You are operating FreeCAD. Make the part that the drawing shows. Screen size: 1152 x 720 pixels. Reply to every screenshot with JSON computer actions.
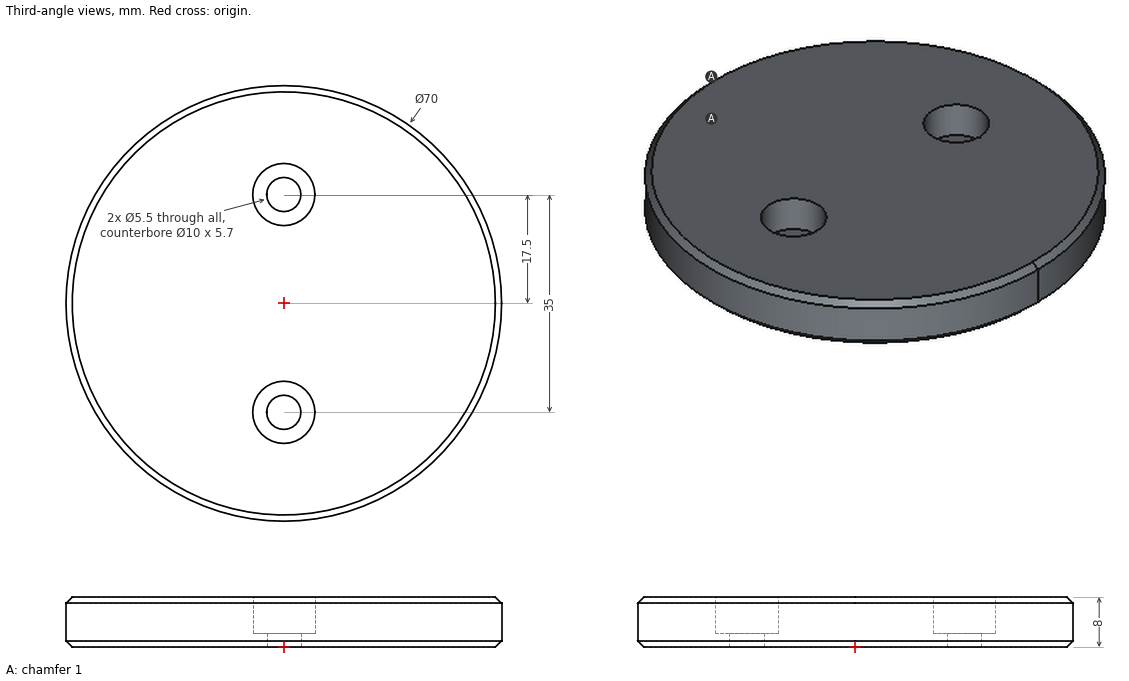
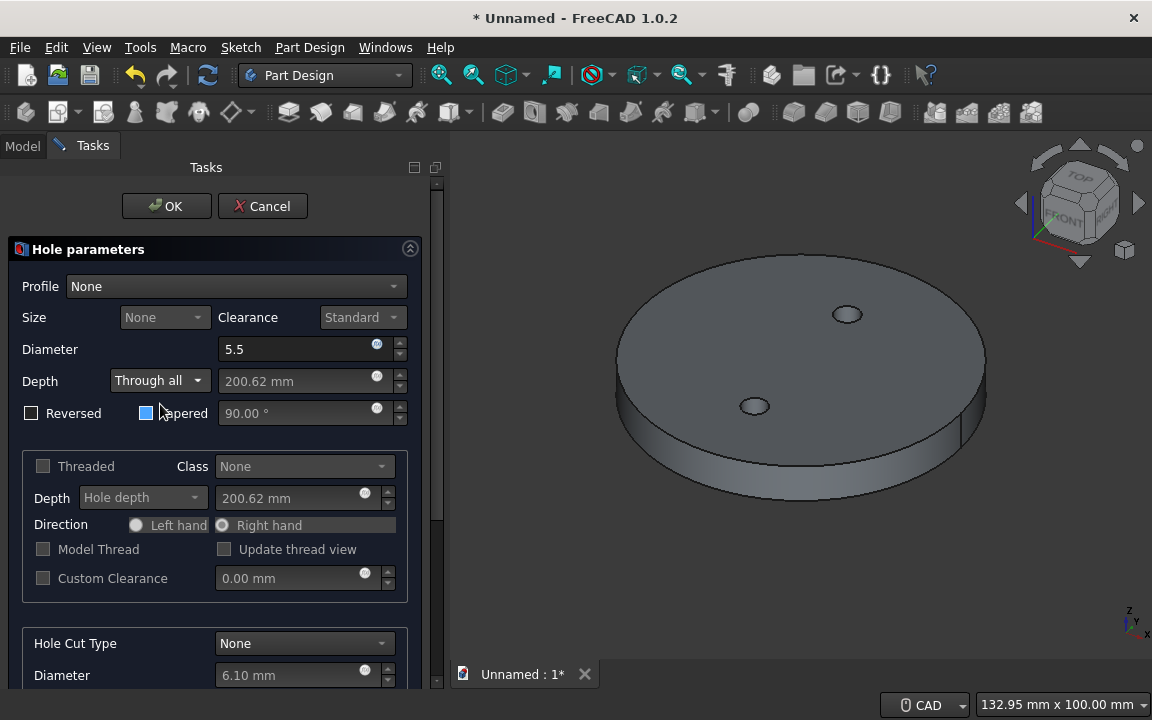
{"action": "left_click", "coordinate": [306, 644]}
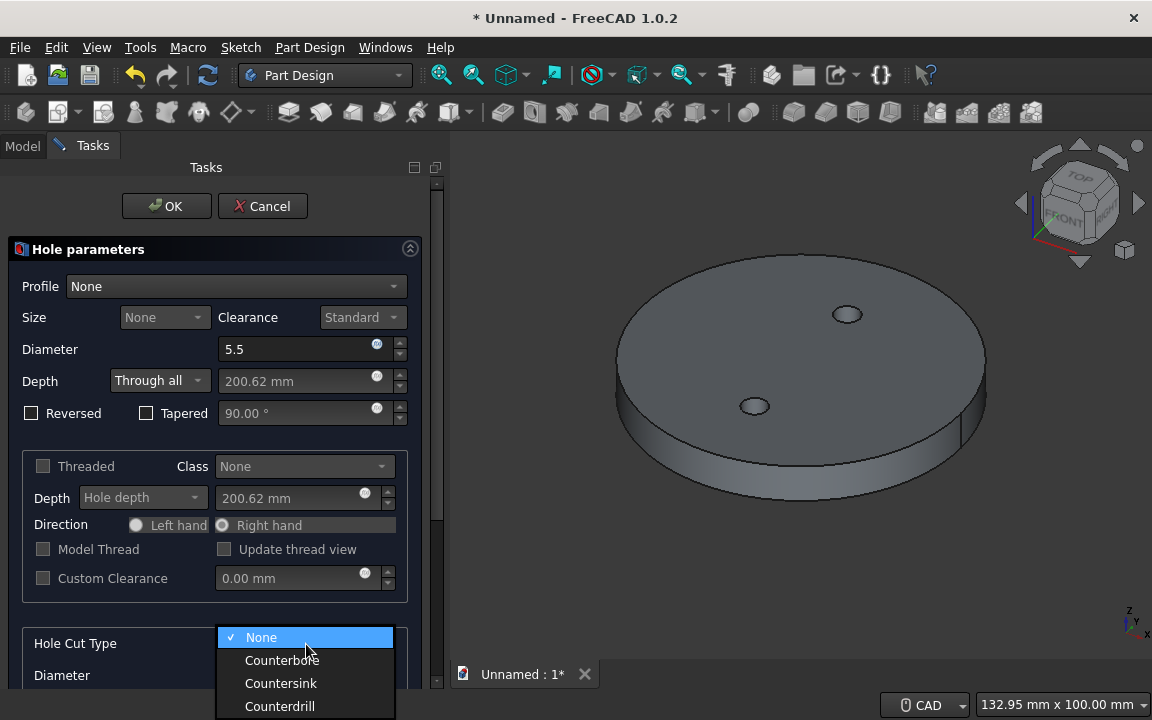
{"action": "left_click", "coordinate": [304, 660]}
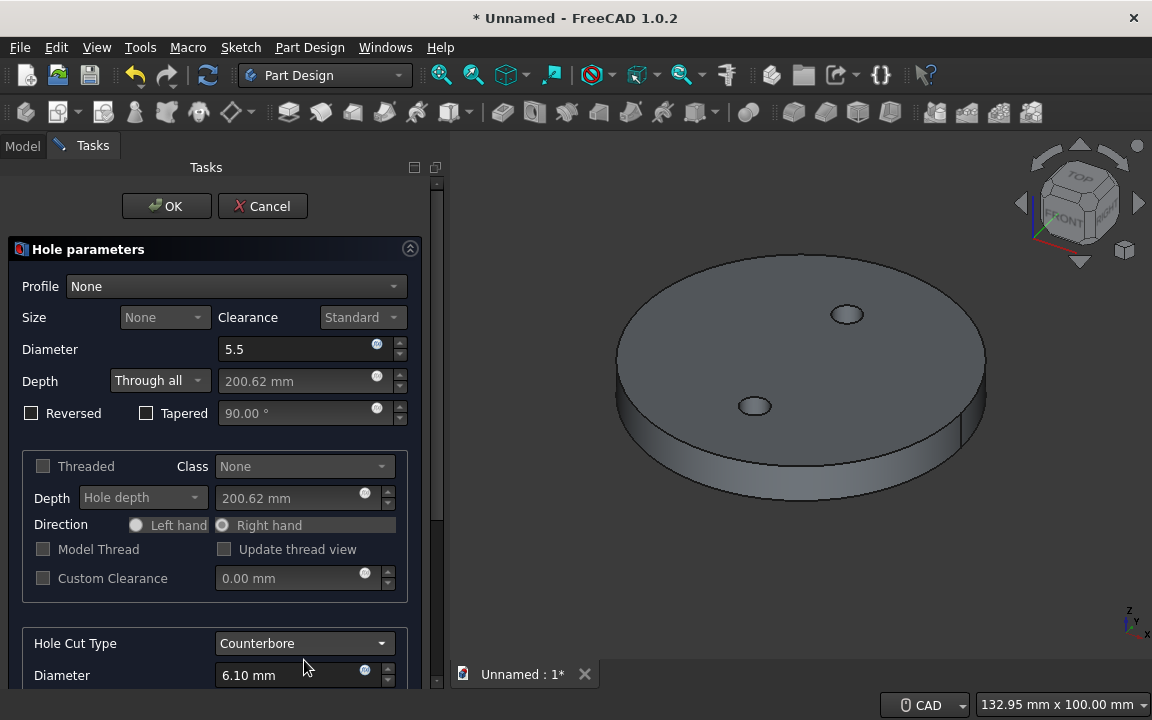
{"action": "triple_click", "coordinate": [298, 675]}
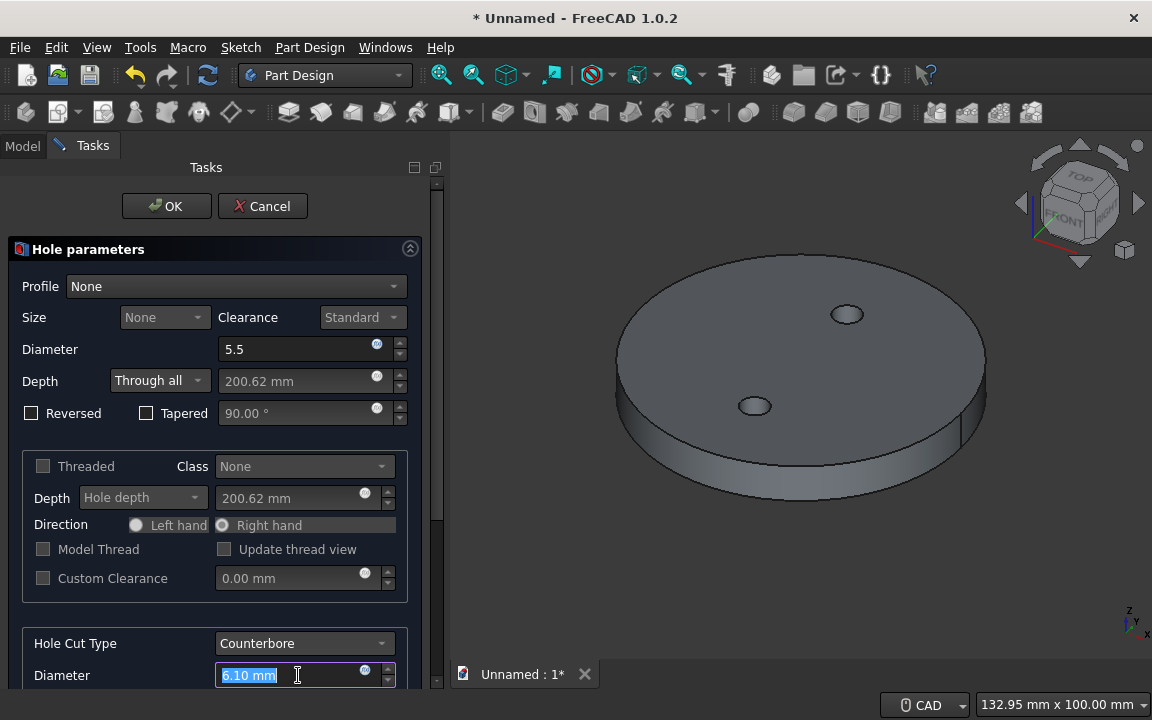
{"action": "type", "text": "10"}
{"action": "key", "text": "Tab"}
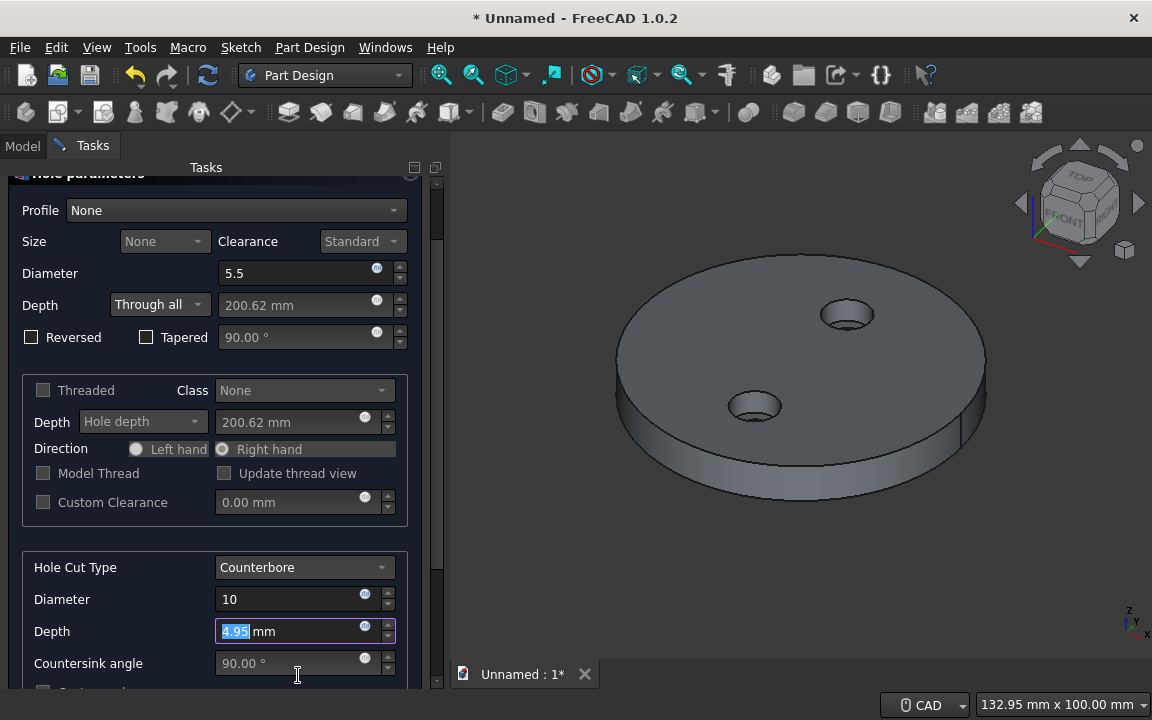
{"action": "type", "text": "5.7"}
{"action": "key", "text": "Tab"}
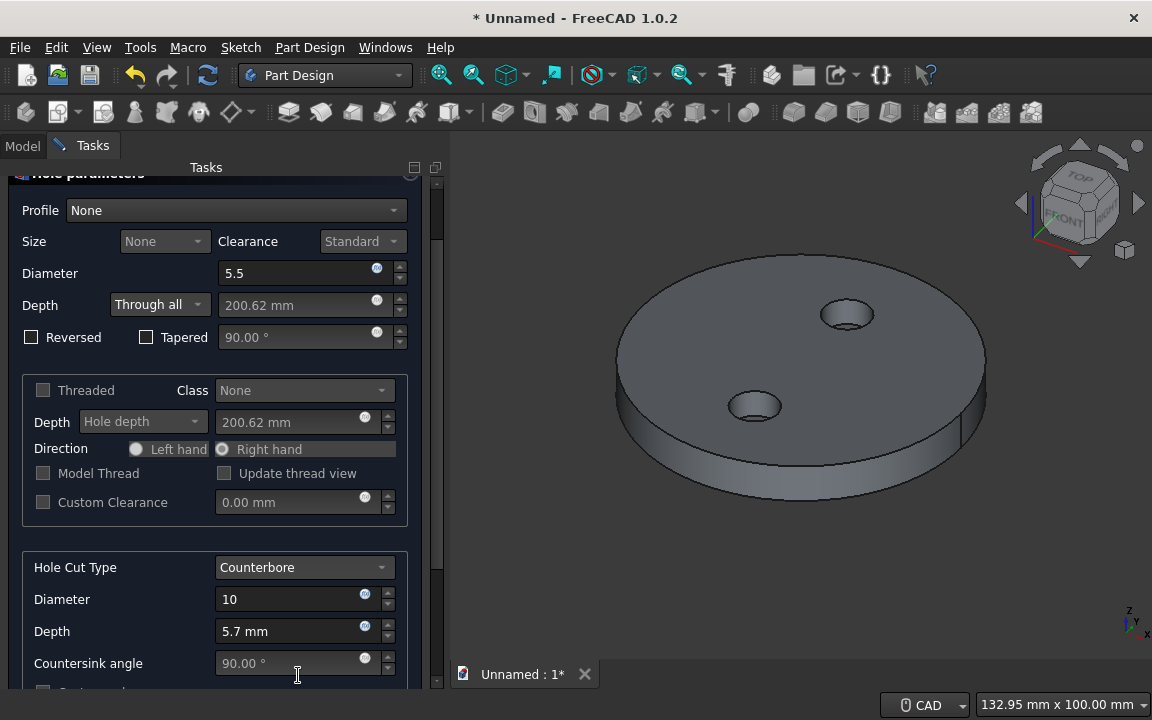
{"action": "scroll", "coordinate": [437, 432], "scroll_direction": "up", "scroll_amount": 3}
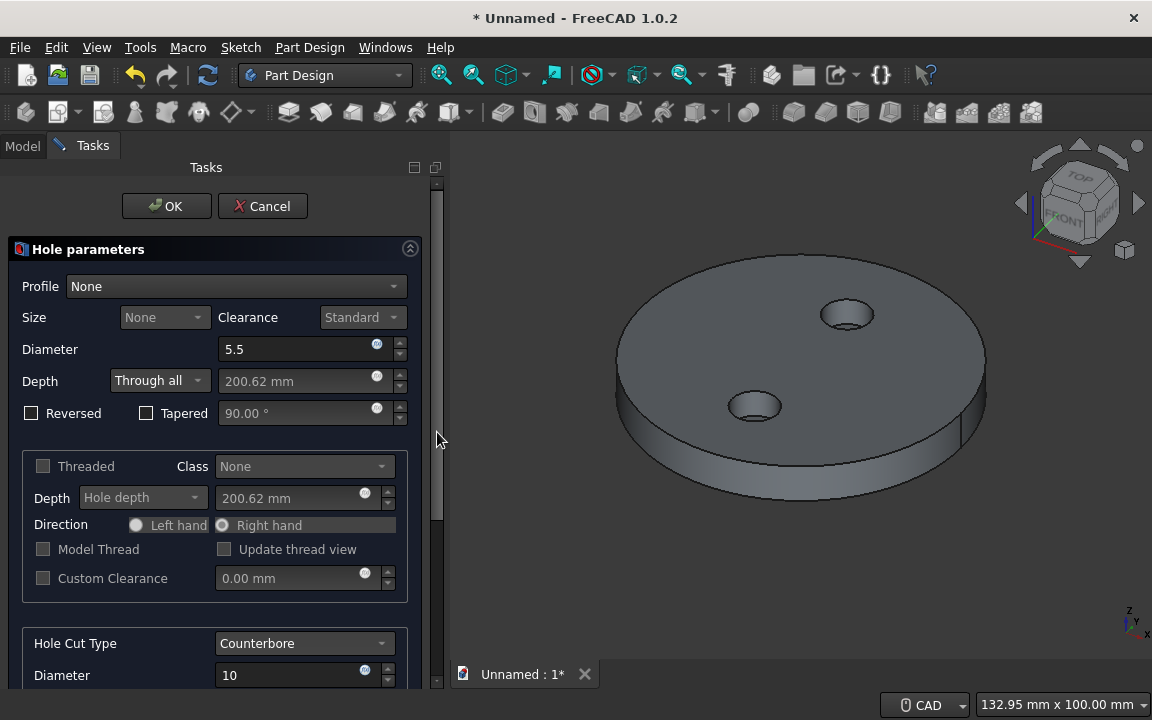
{"action": "left_click", "coordinate": [167, 206]}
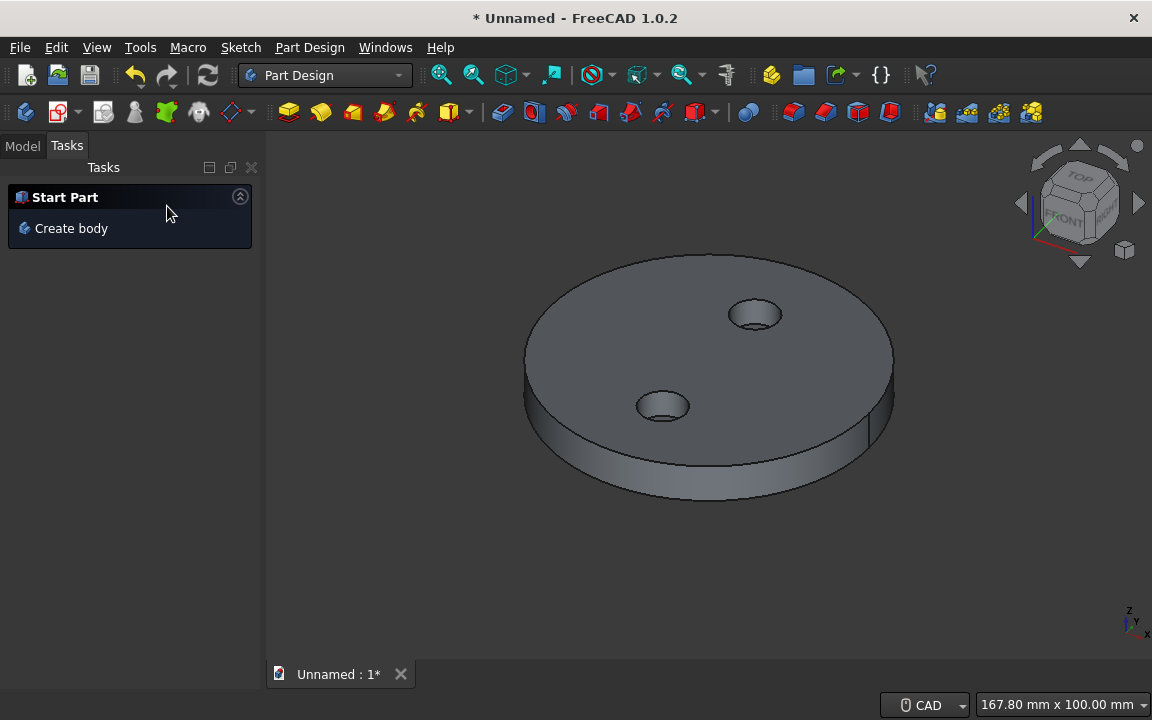
{"action": "left_click", "coordinate": [525, 370]}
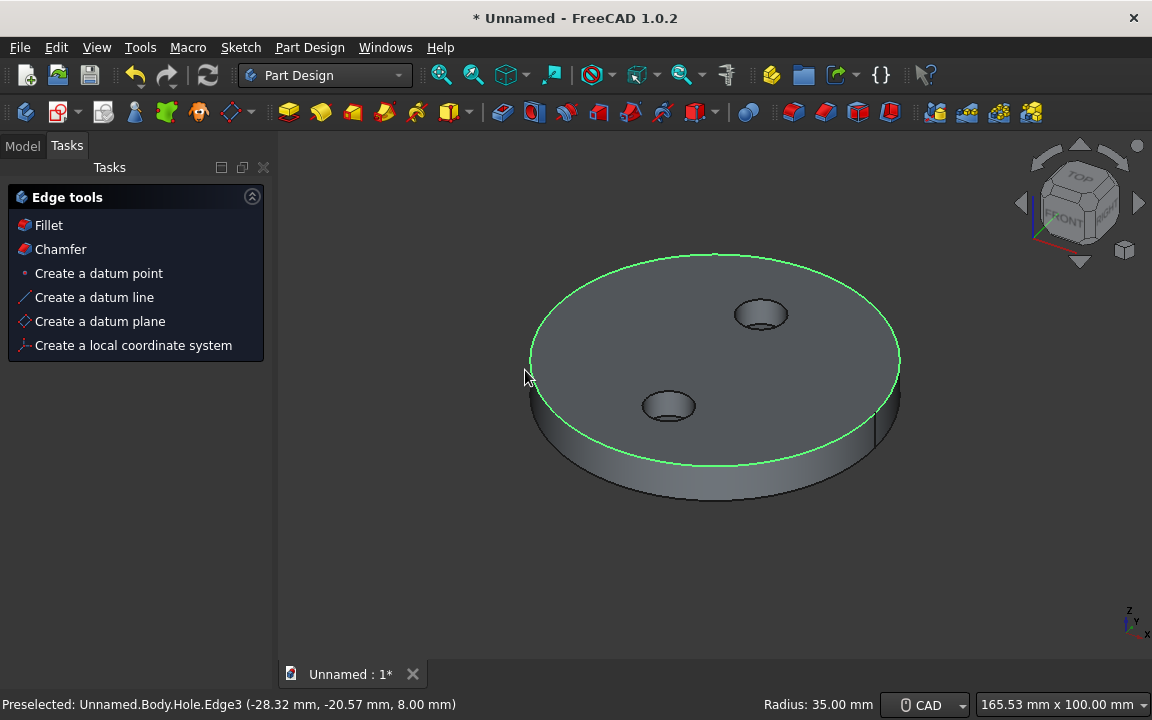
{"action": "key", "text": "0"}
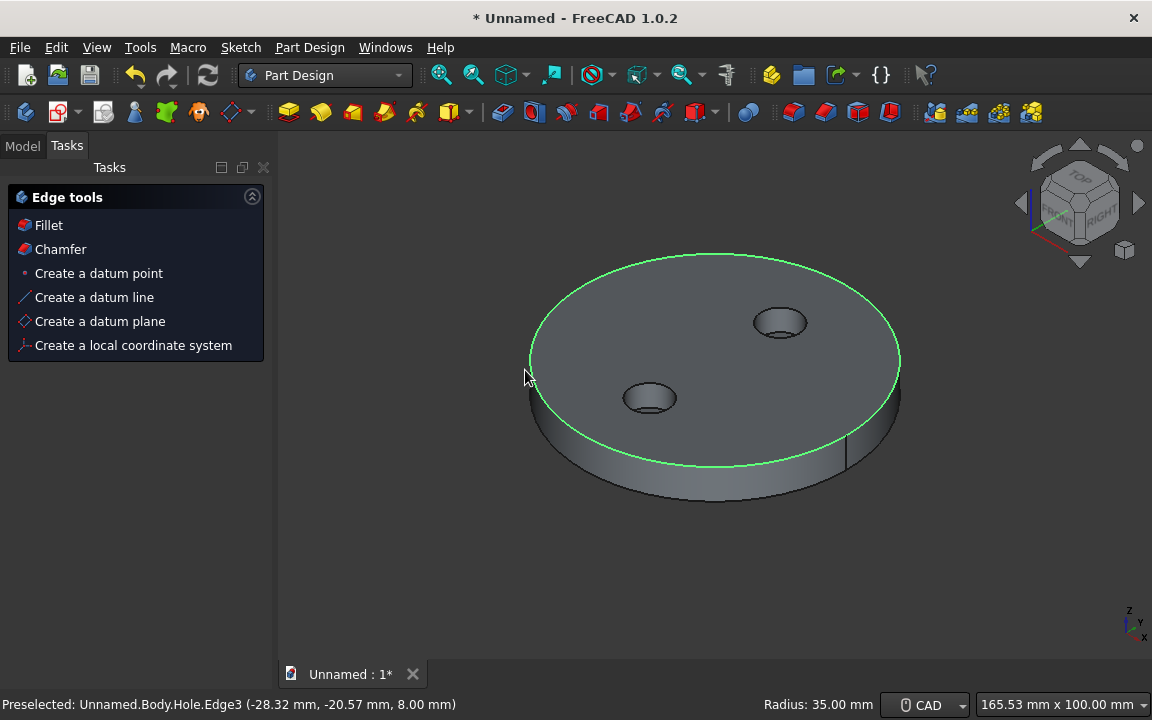
{"action": "key", "text": "2"}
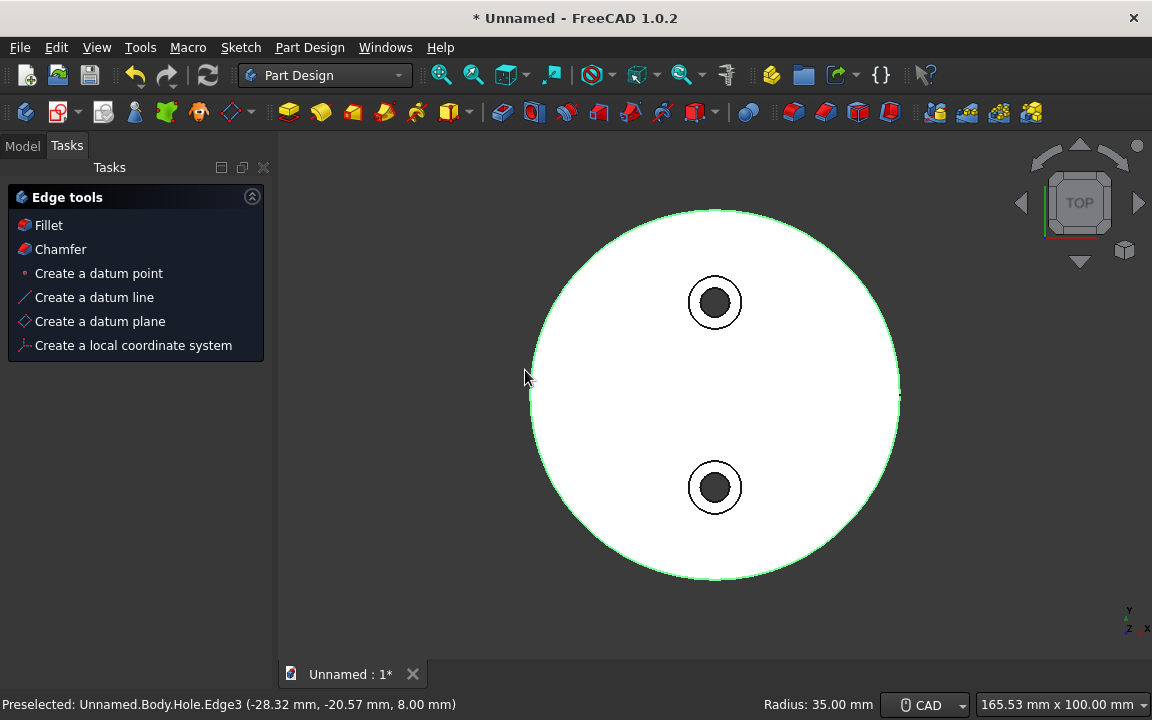
{"action": "key", "text": "1"}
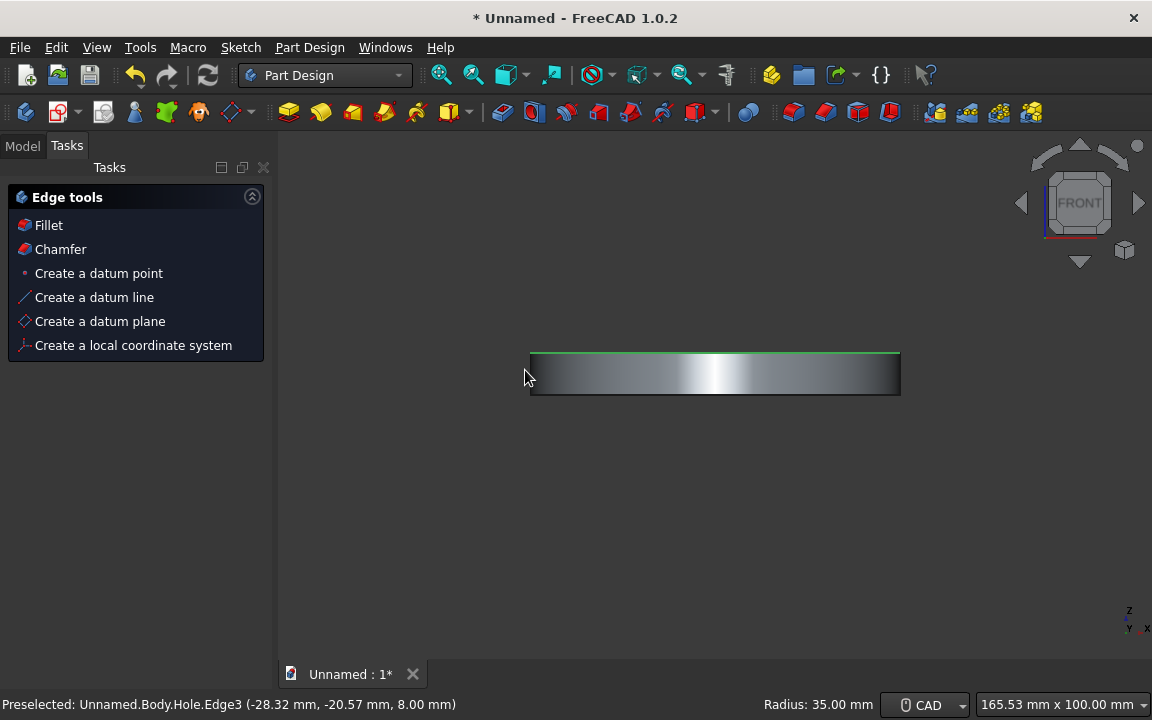
{"action": "left_click", "coordinate": [442, 76]}